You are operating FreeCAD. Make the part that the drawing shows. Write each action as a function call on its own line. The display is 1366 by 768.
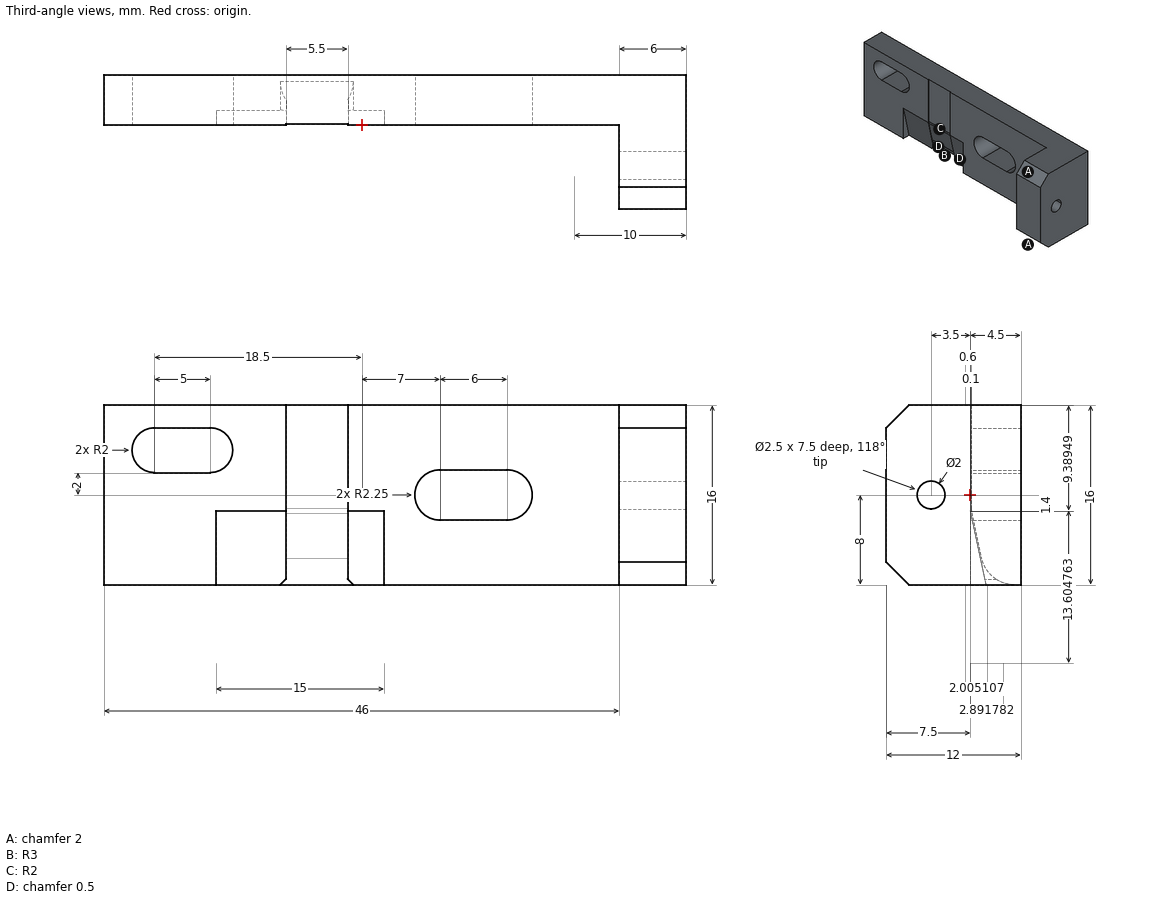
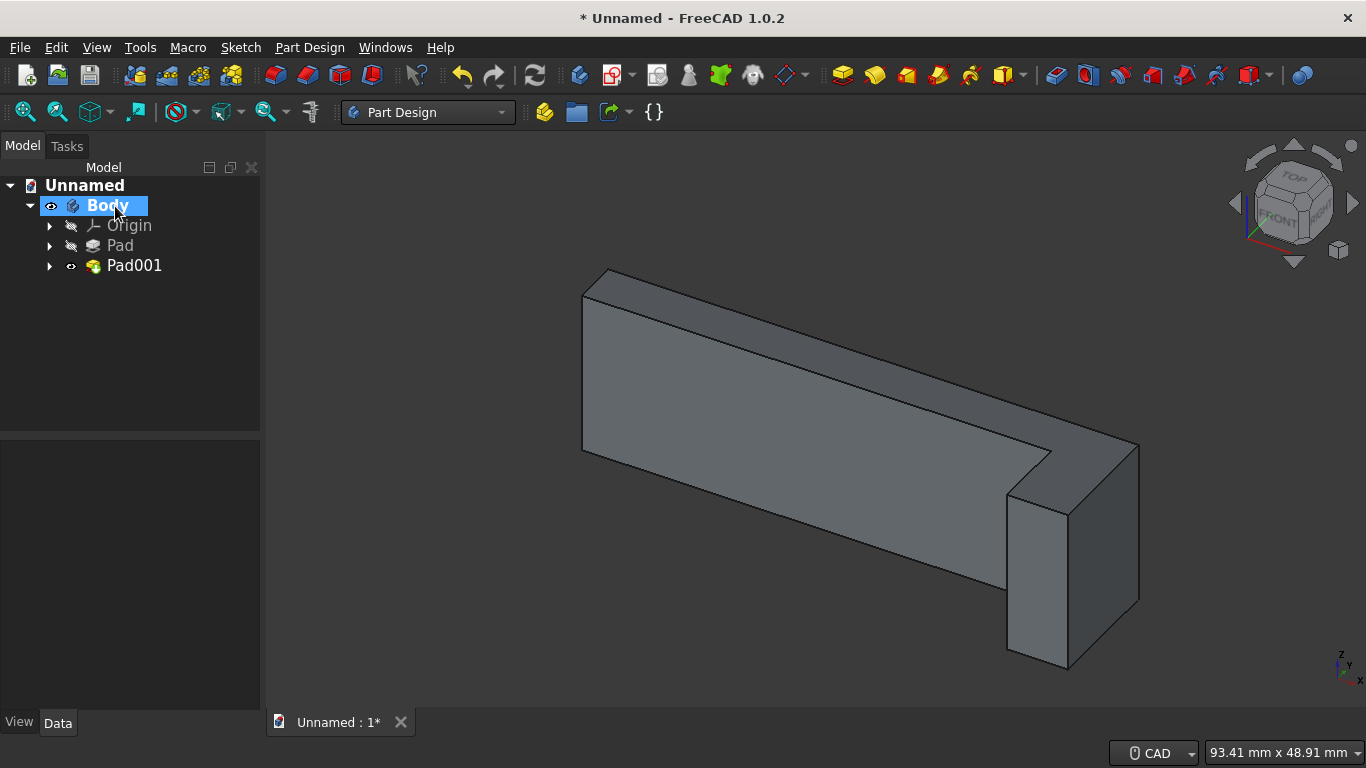
click(1103, 556)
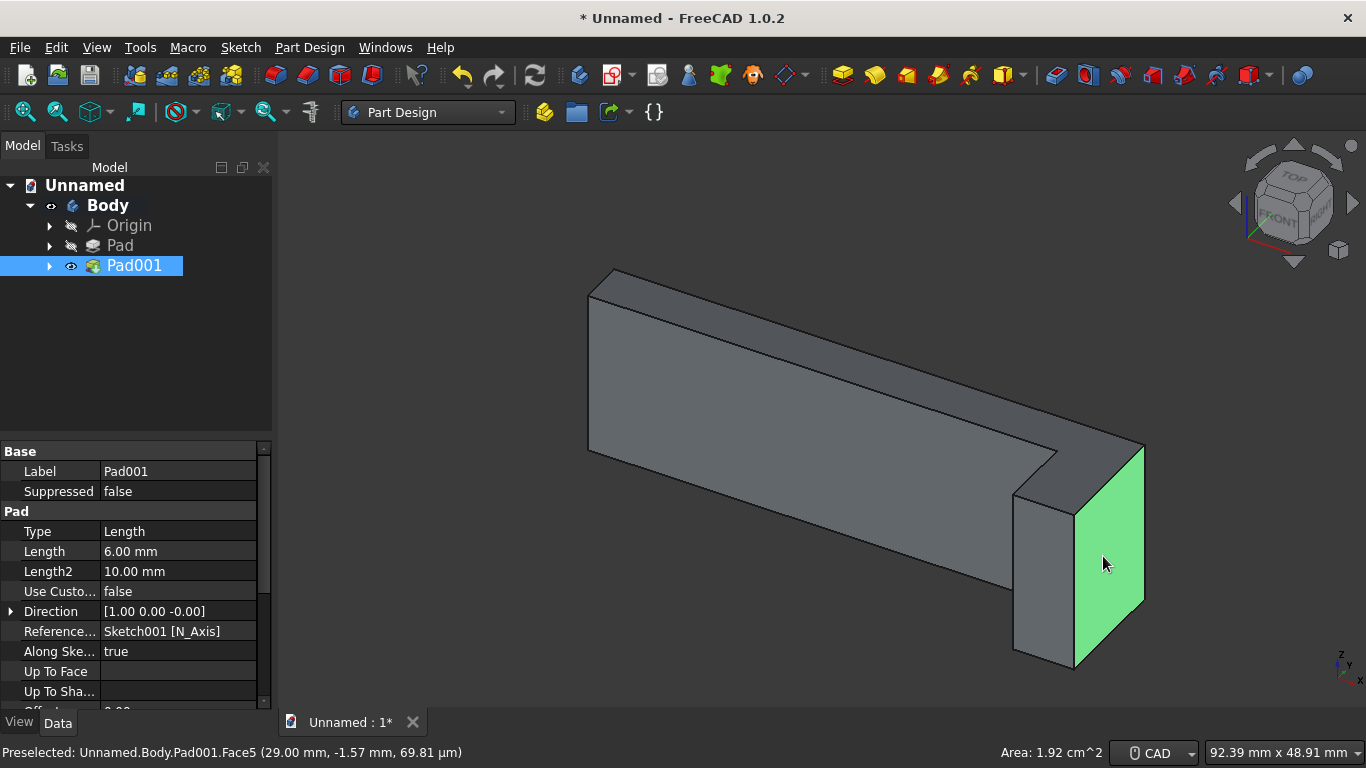
click(612, 76)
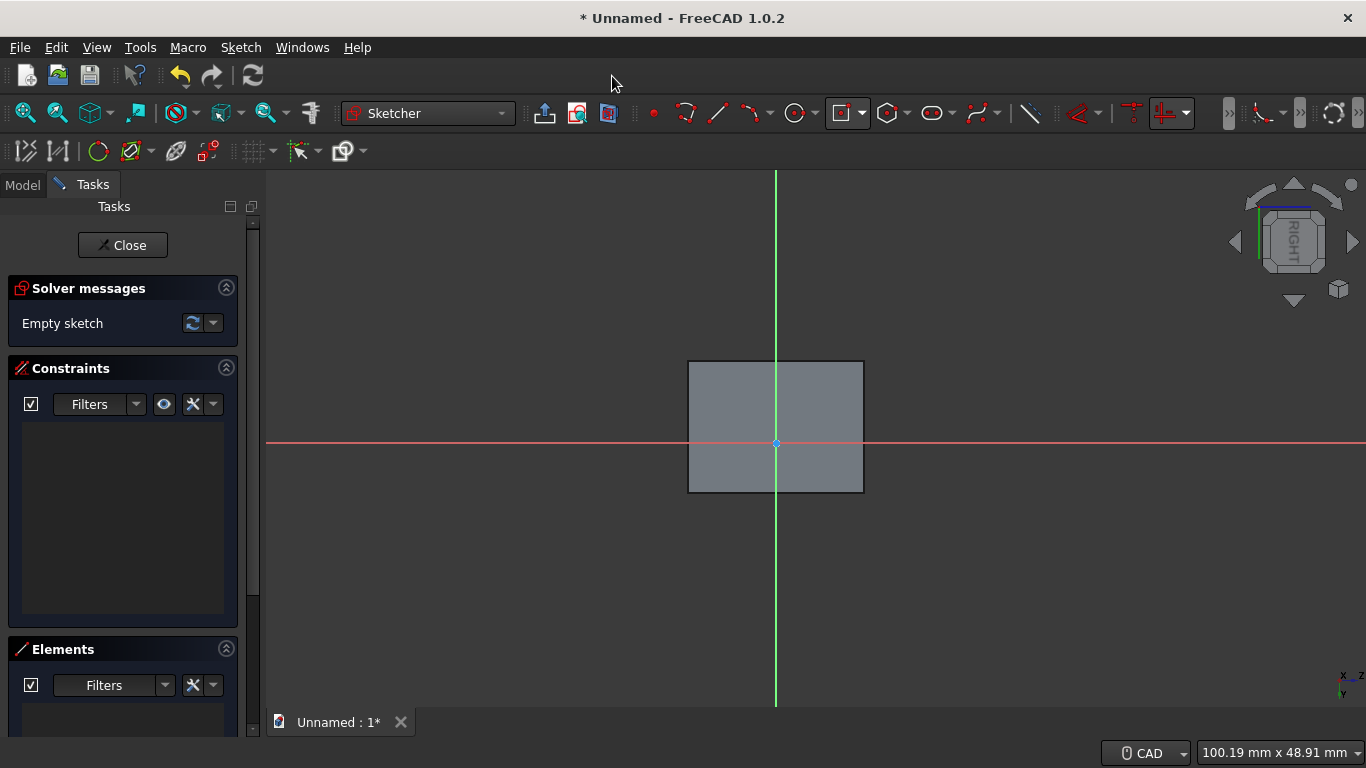
scroll(781, 416, up, 10)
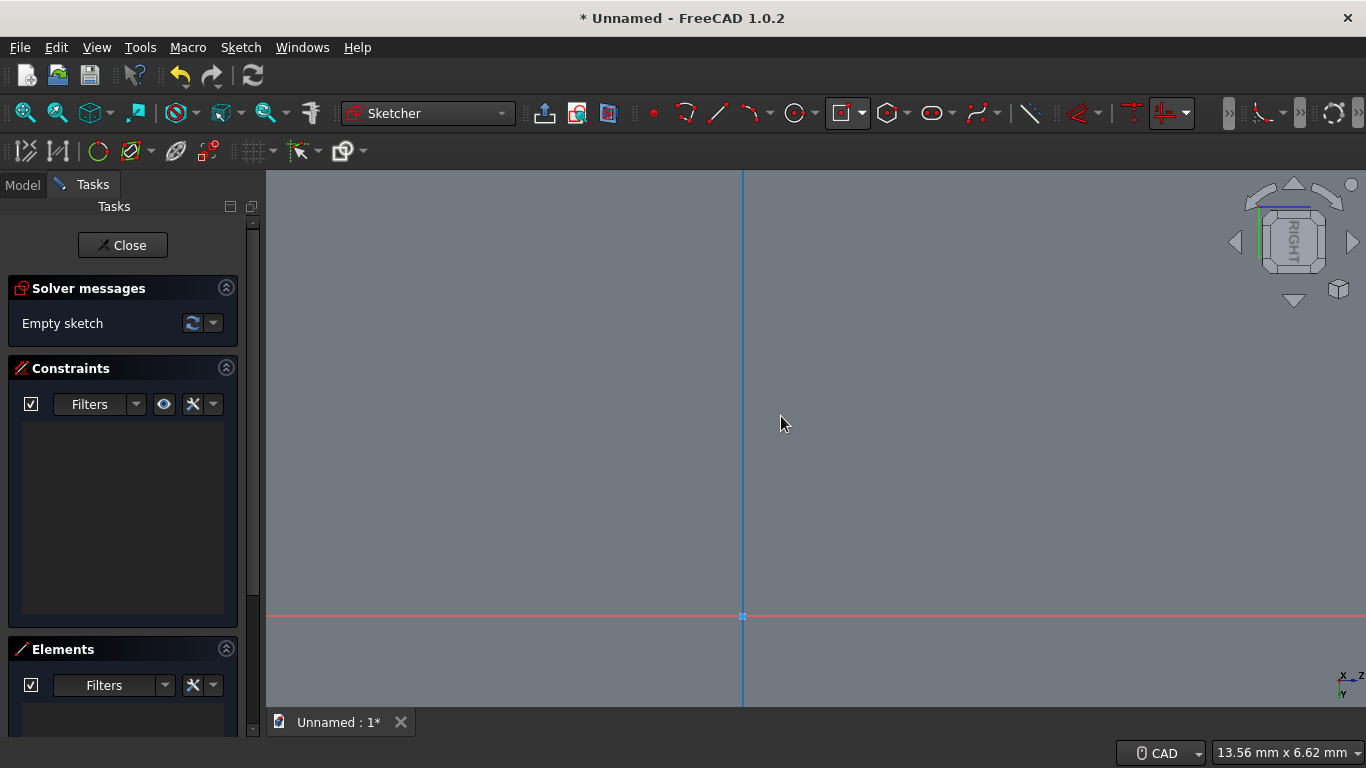
key(g)
key(c)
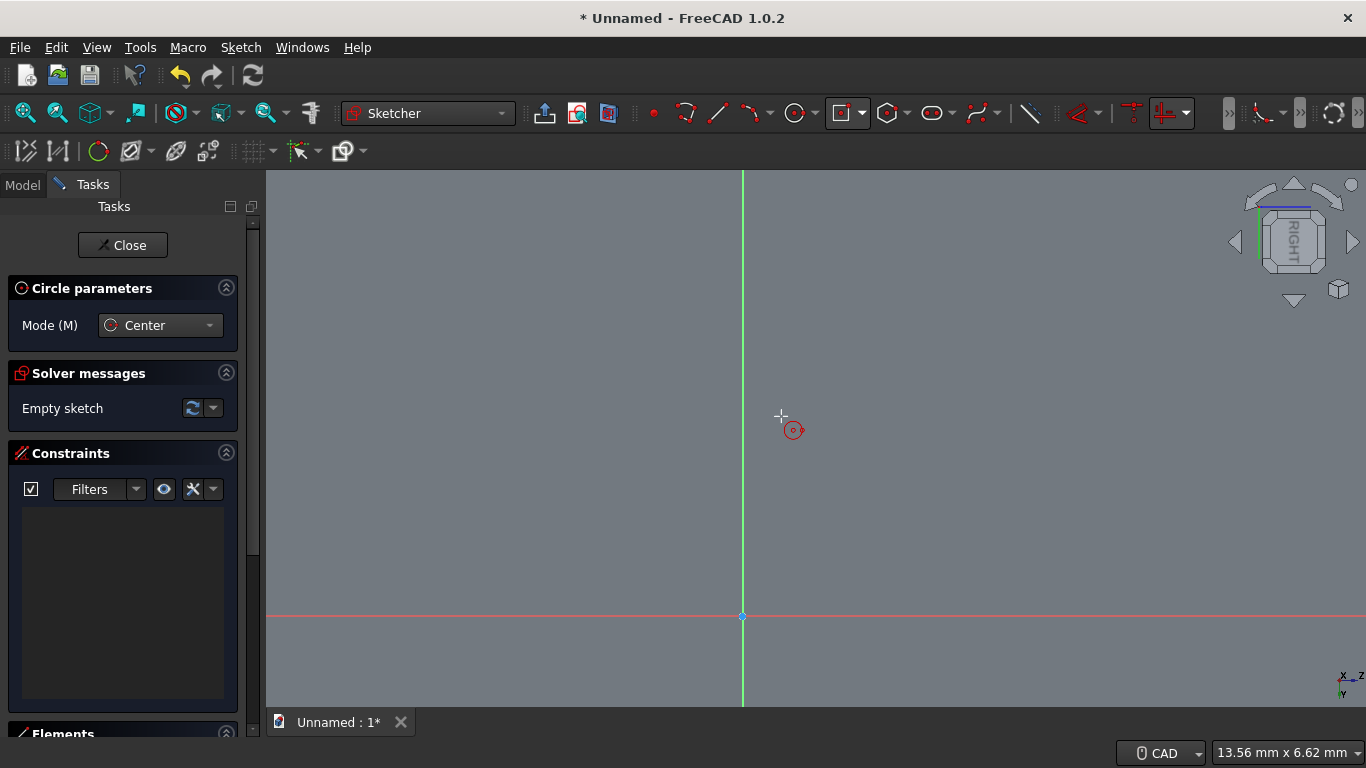
click(743, 332)
click(800, 275)
key(Escape)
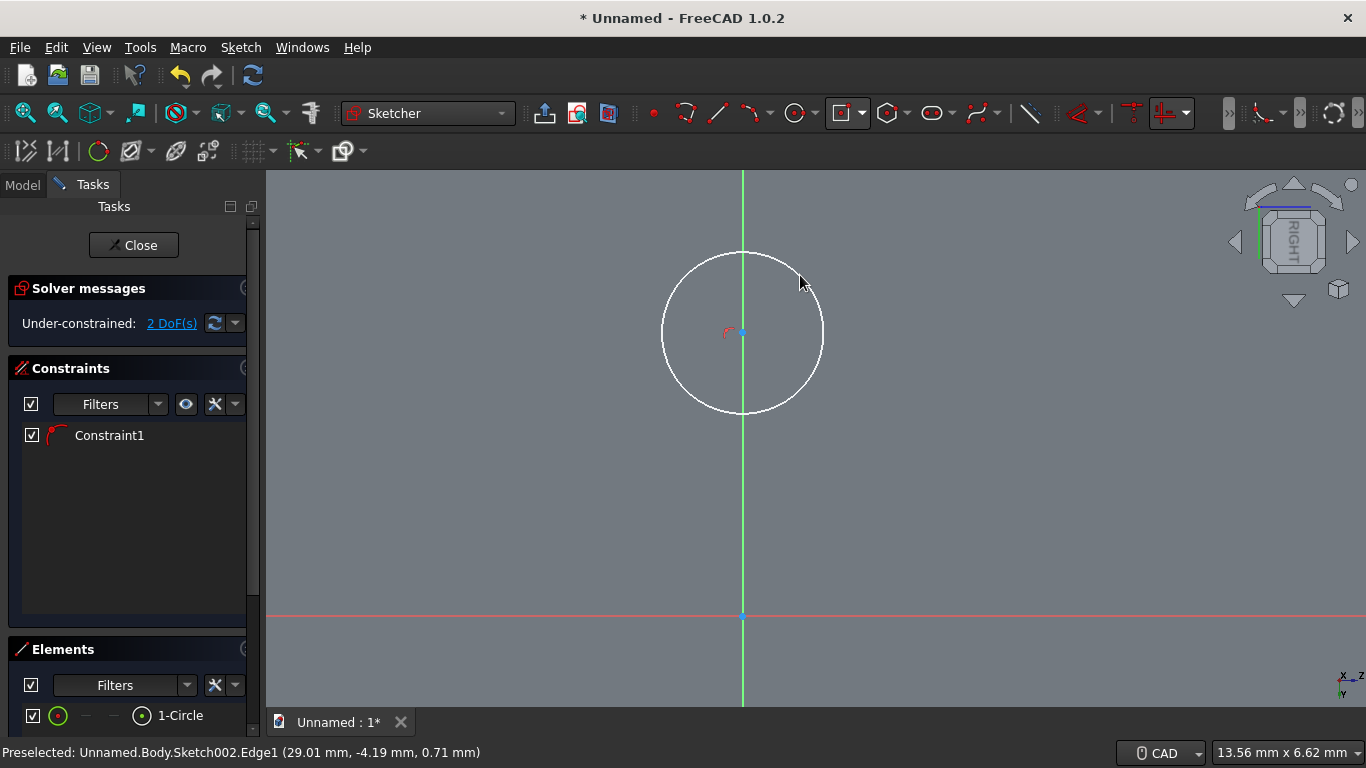
click(1078, 114)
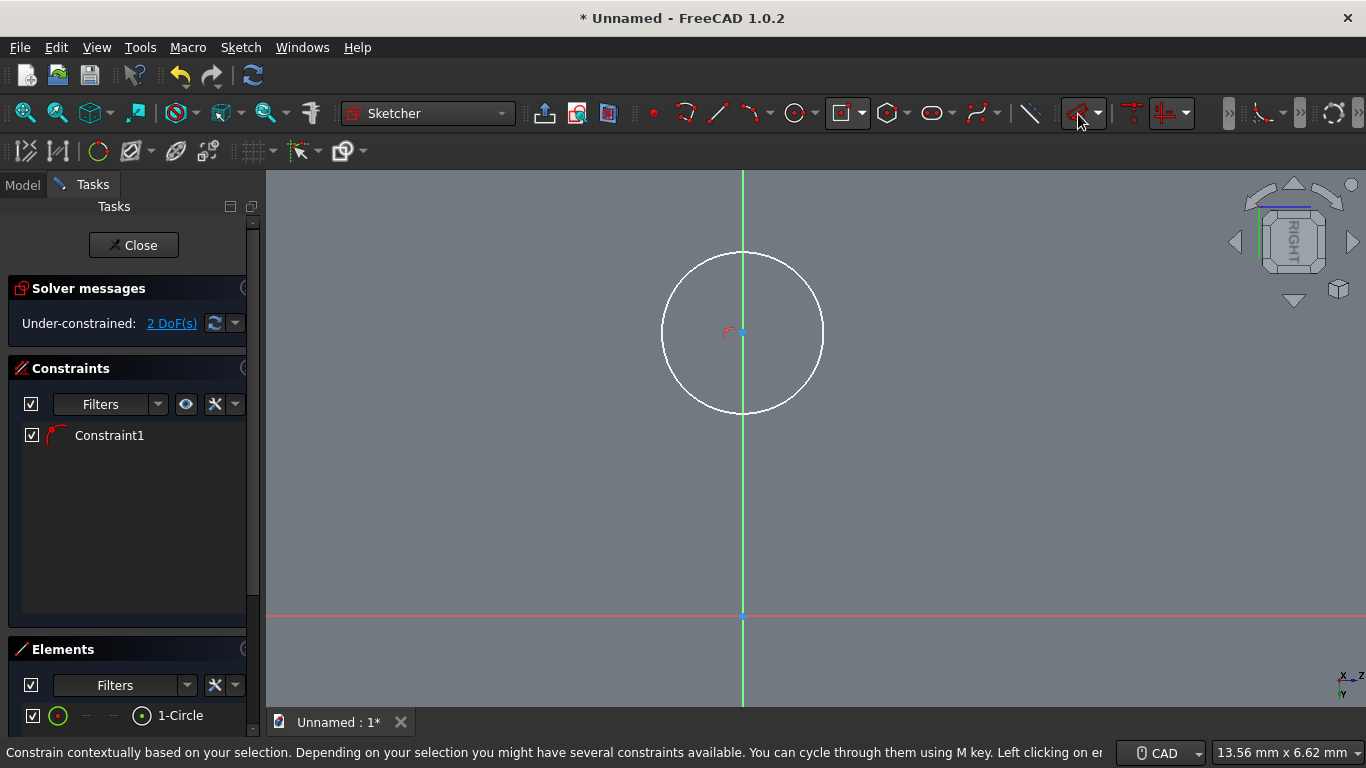
click(800, 276)
click(823, 253)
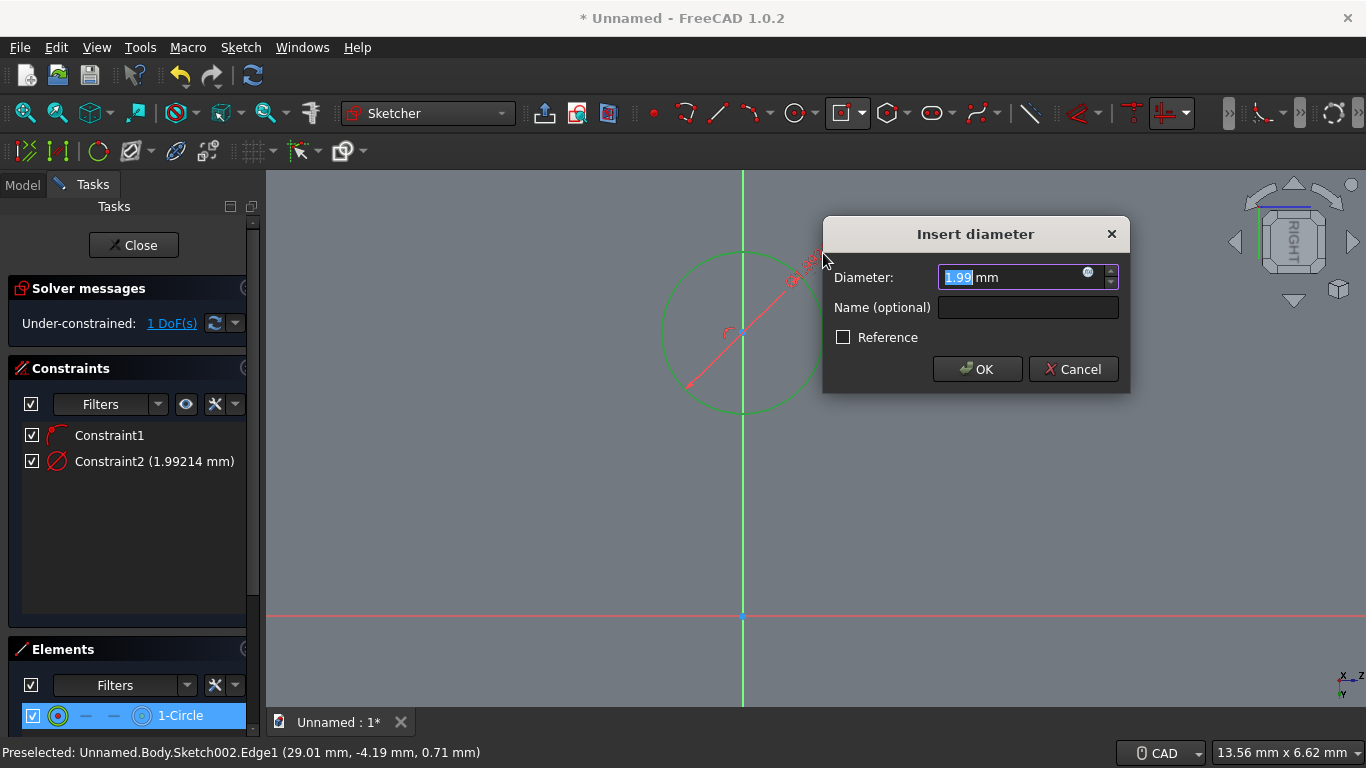
text(2)
key(Return)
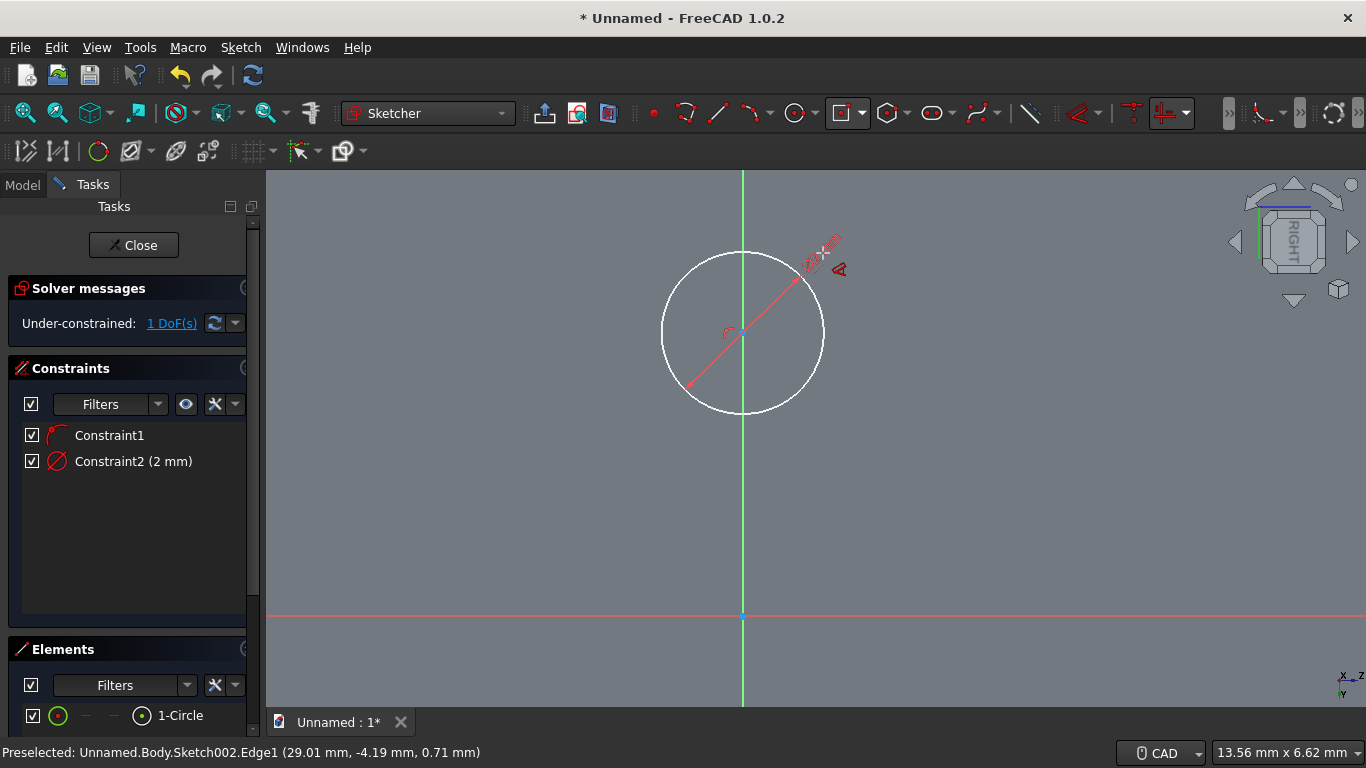
click(745, 335)
click(777, 475)